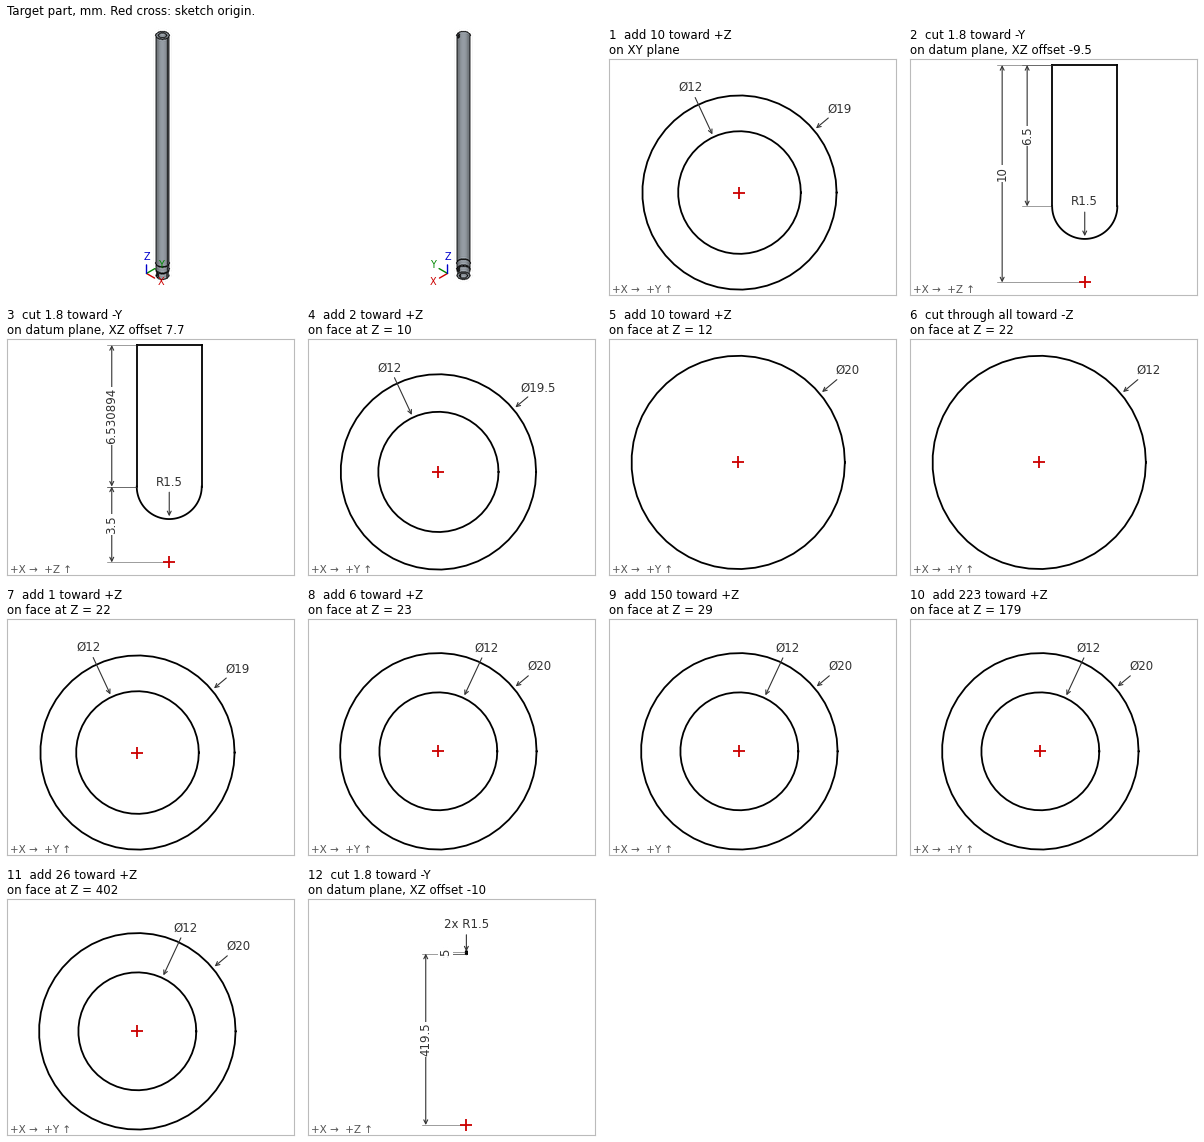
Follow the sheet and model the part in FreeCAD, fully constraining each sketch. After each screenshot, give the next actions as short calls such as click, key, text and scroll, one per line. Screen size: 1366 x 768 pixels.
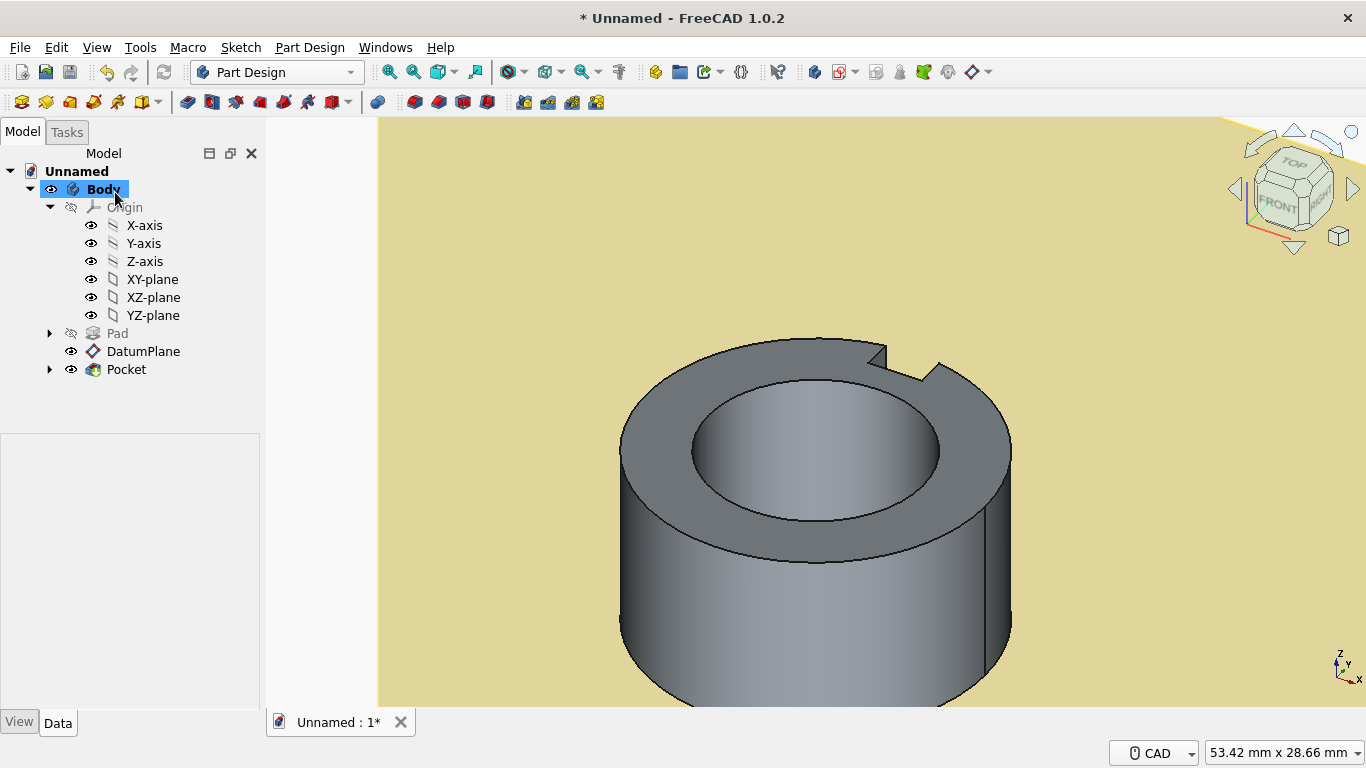
click(116, 351)
key(space)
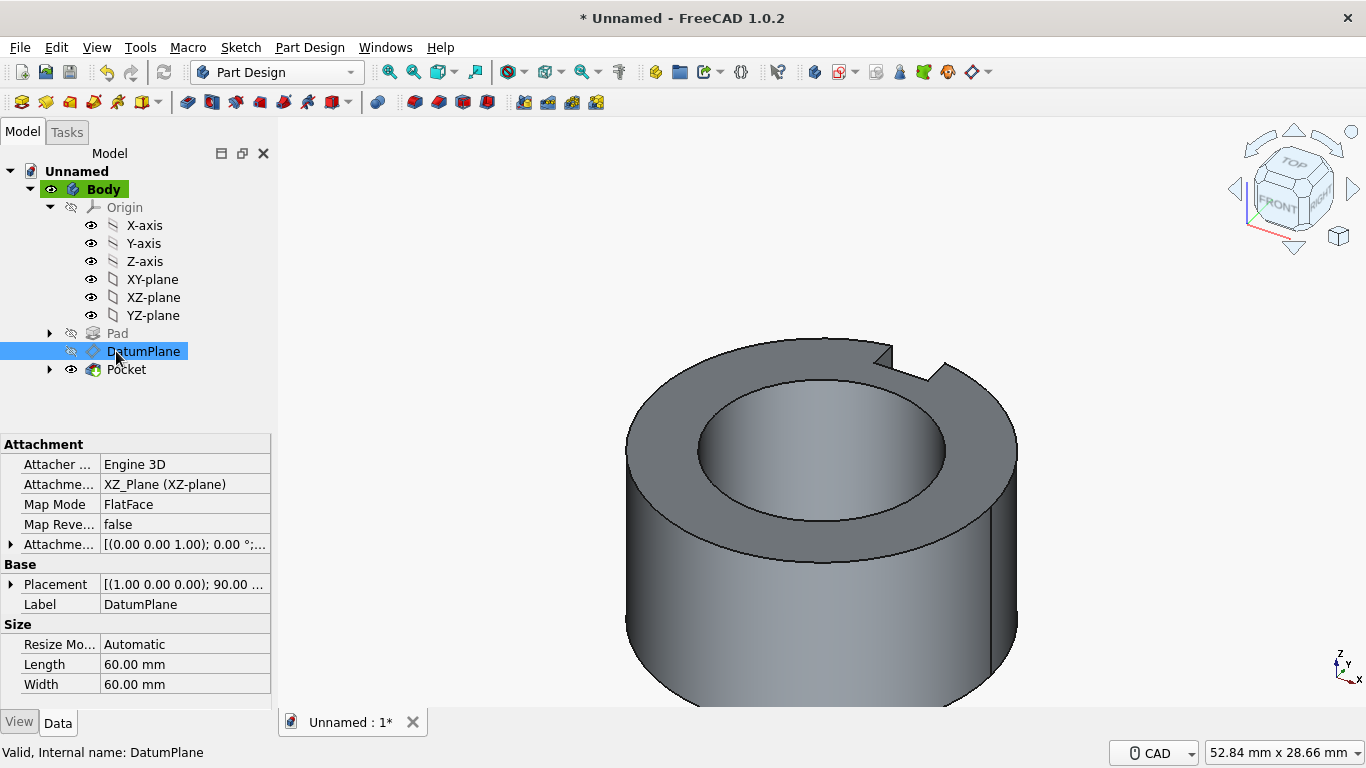
click(390, 72)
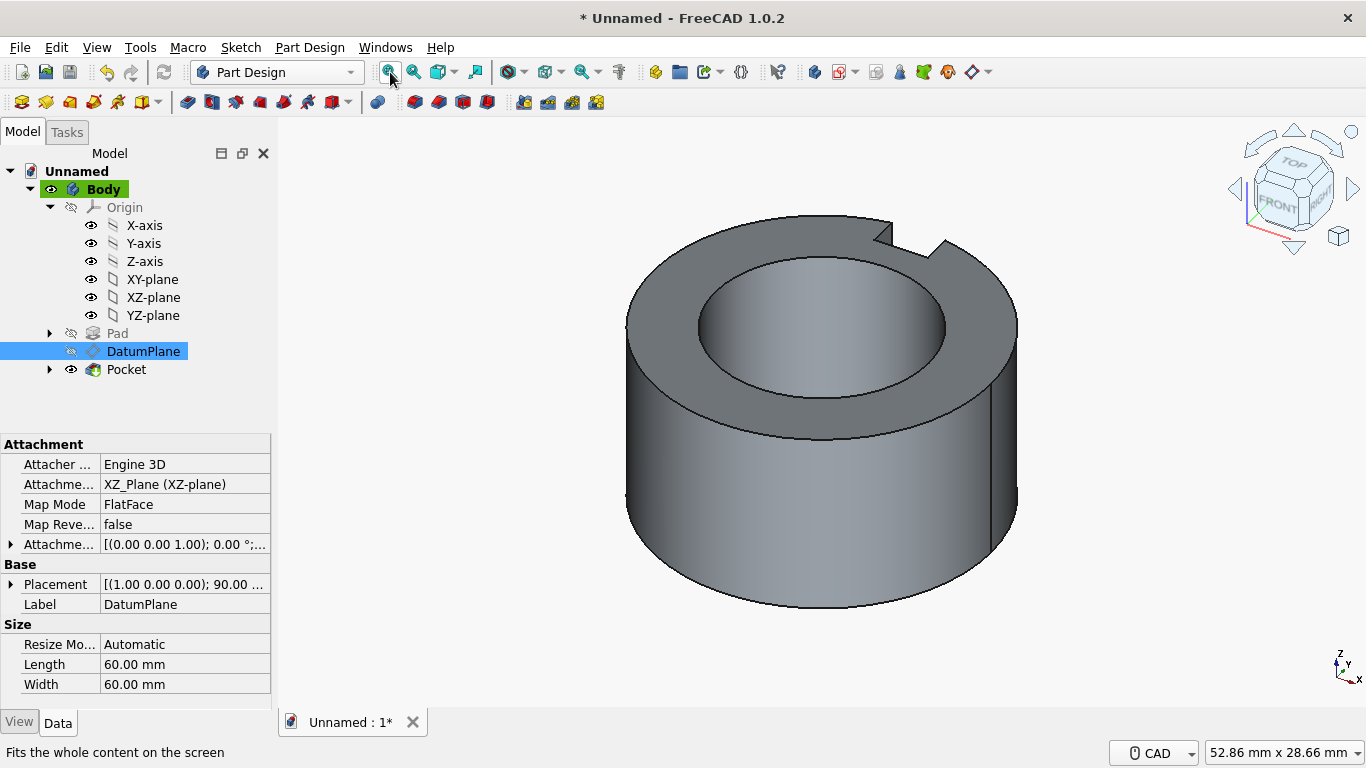
click(136, 297)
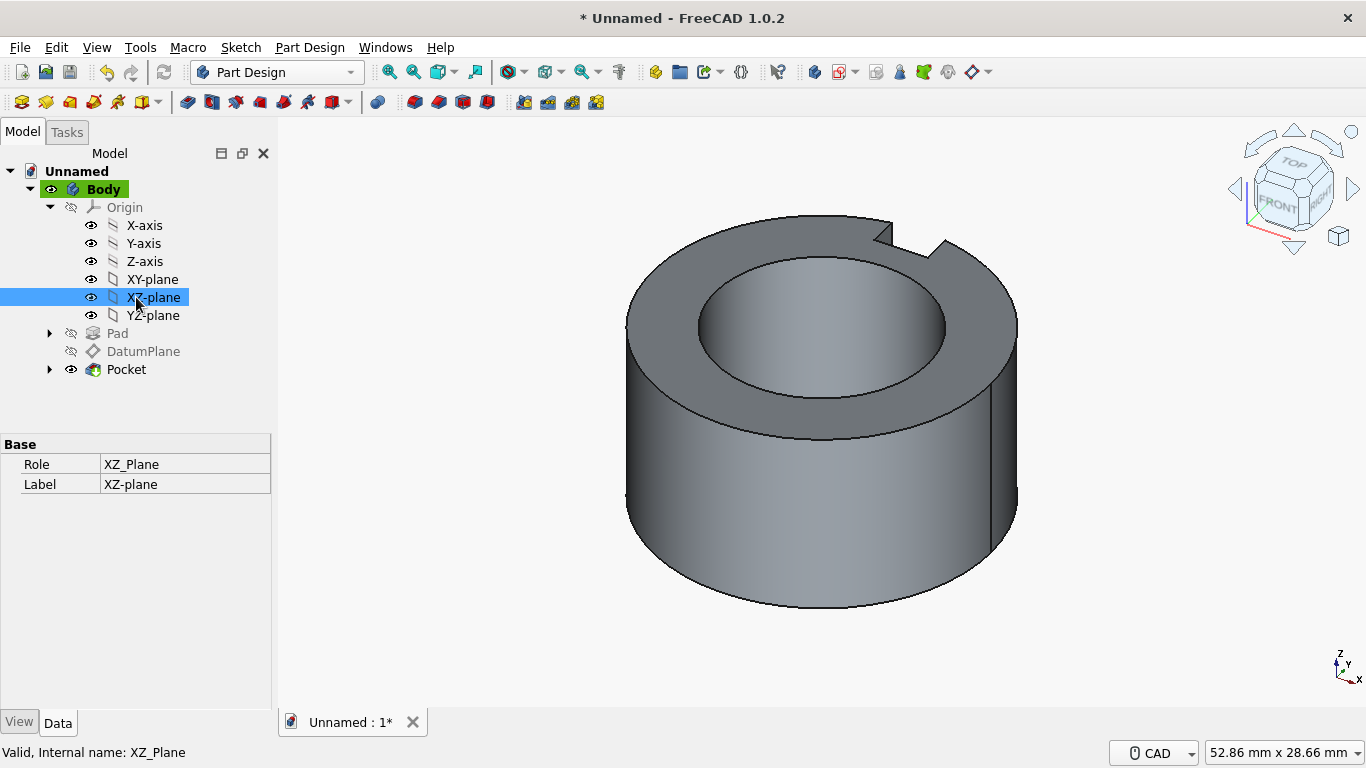
click(972, 72)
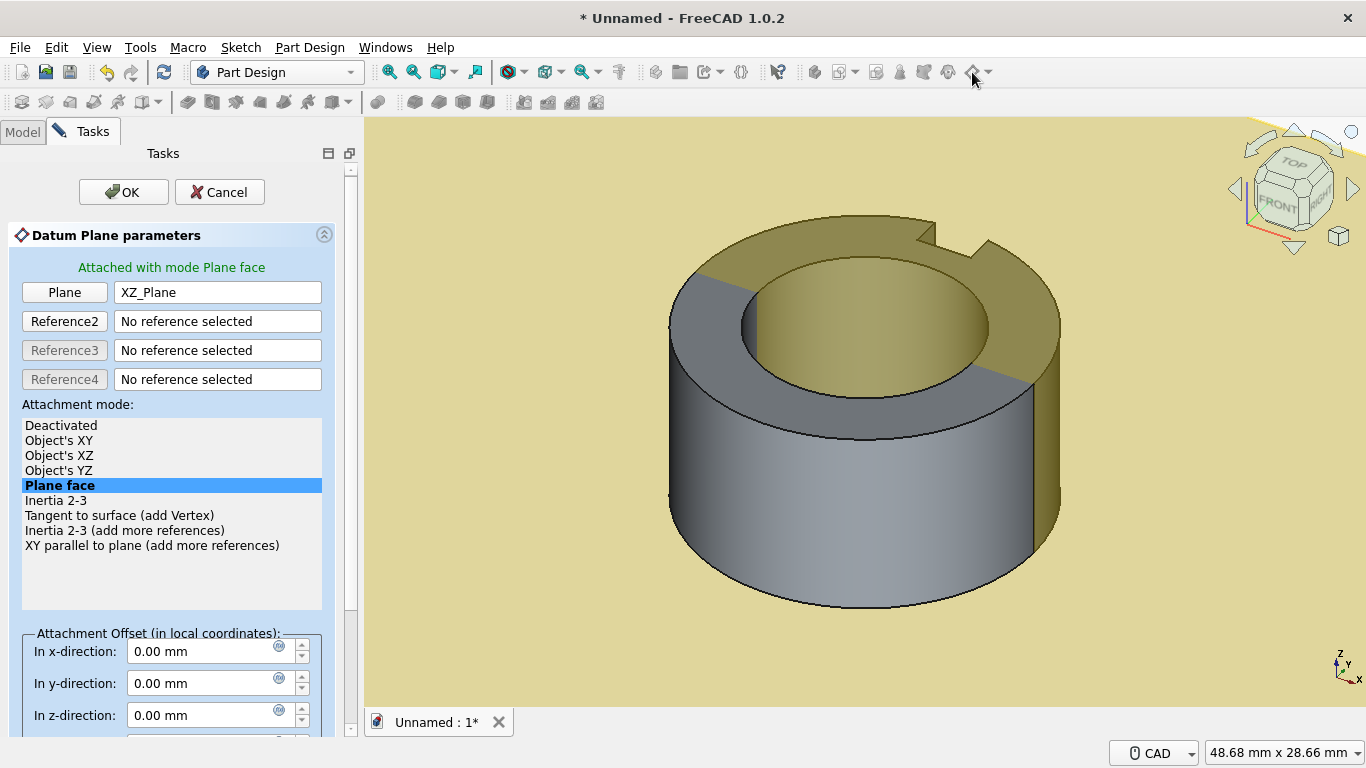
triple_click(210, 715)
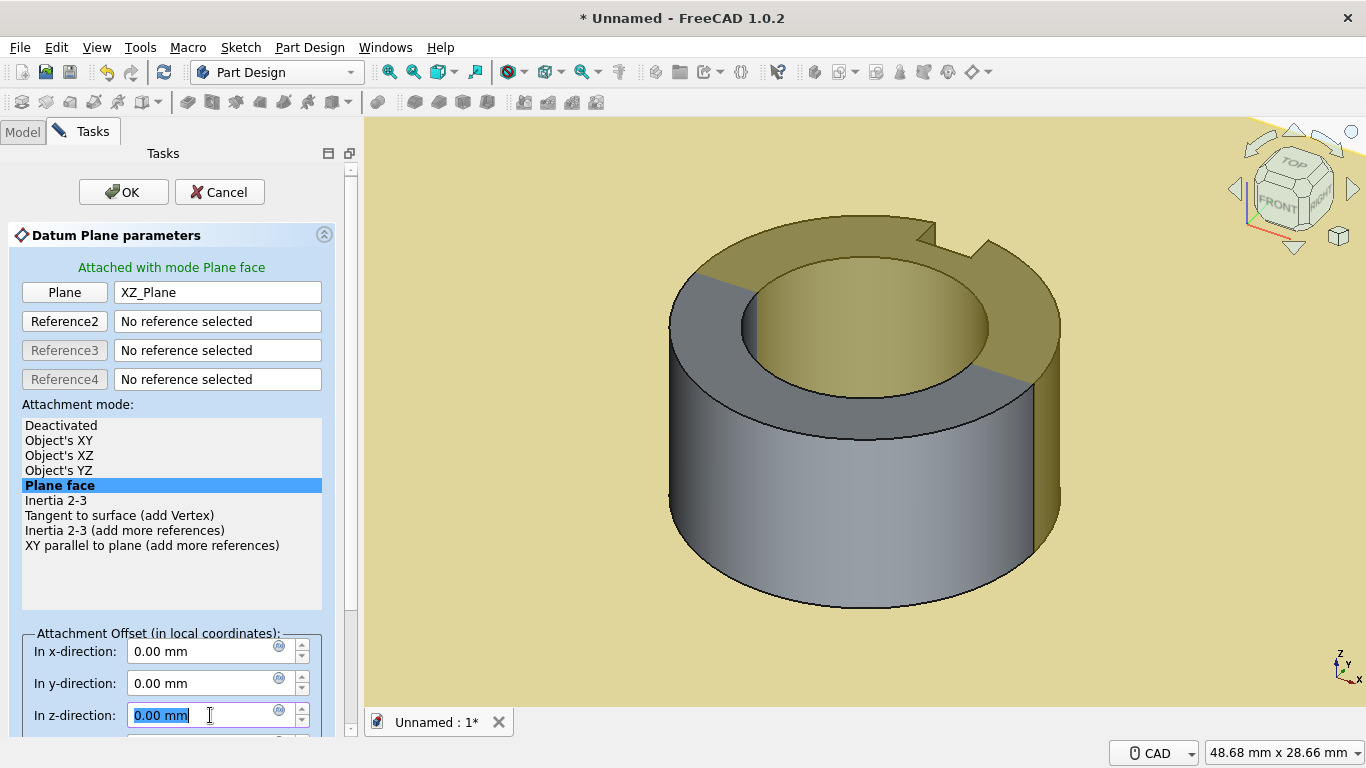
text(7.7)
key(Tab)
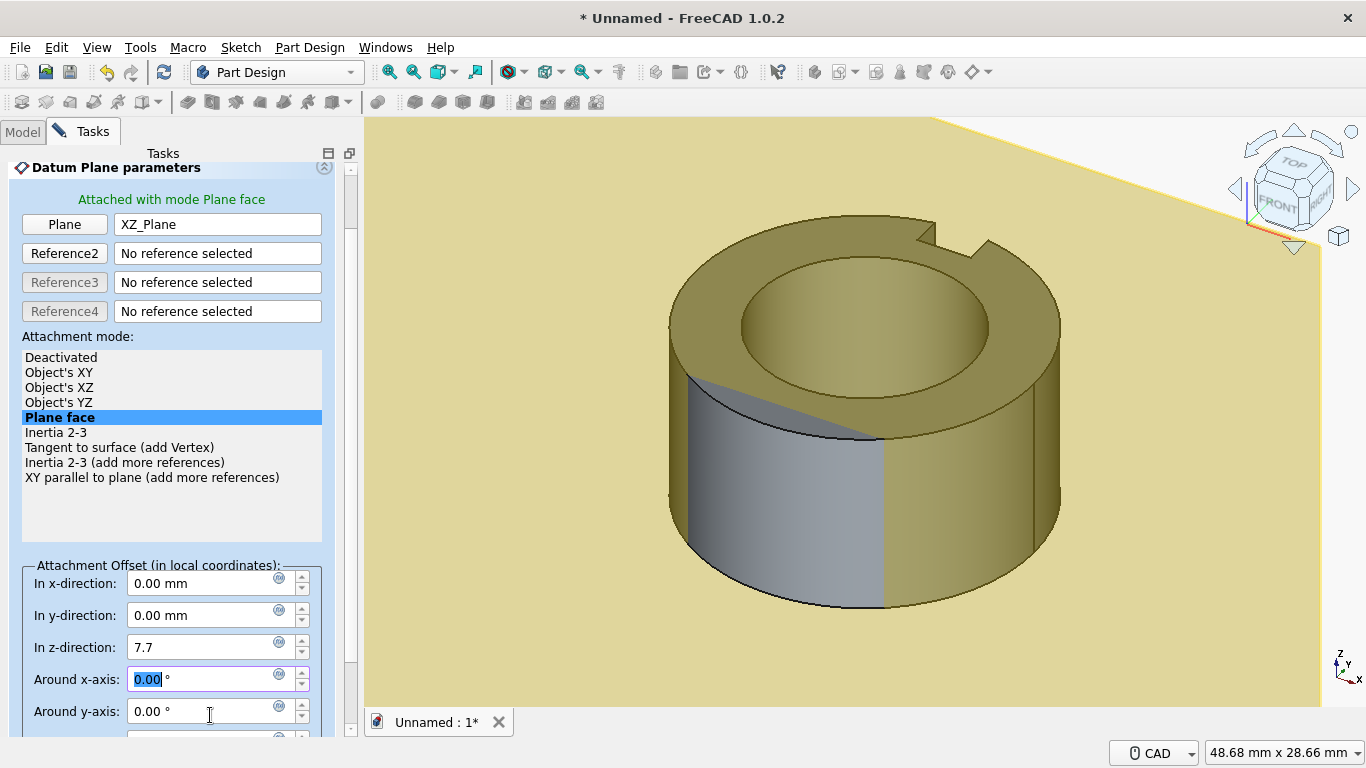
scroll(351, 450, up, 2)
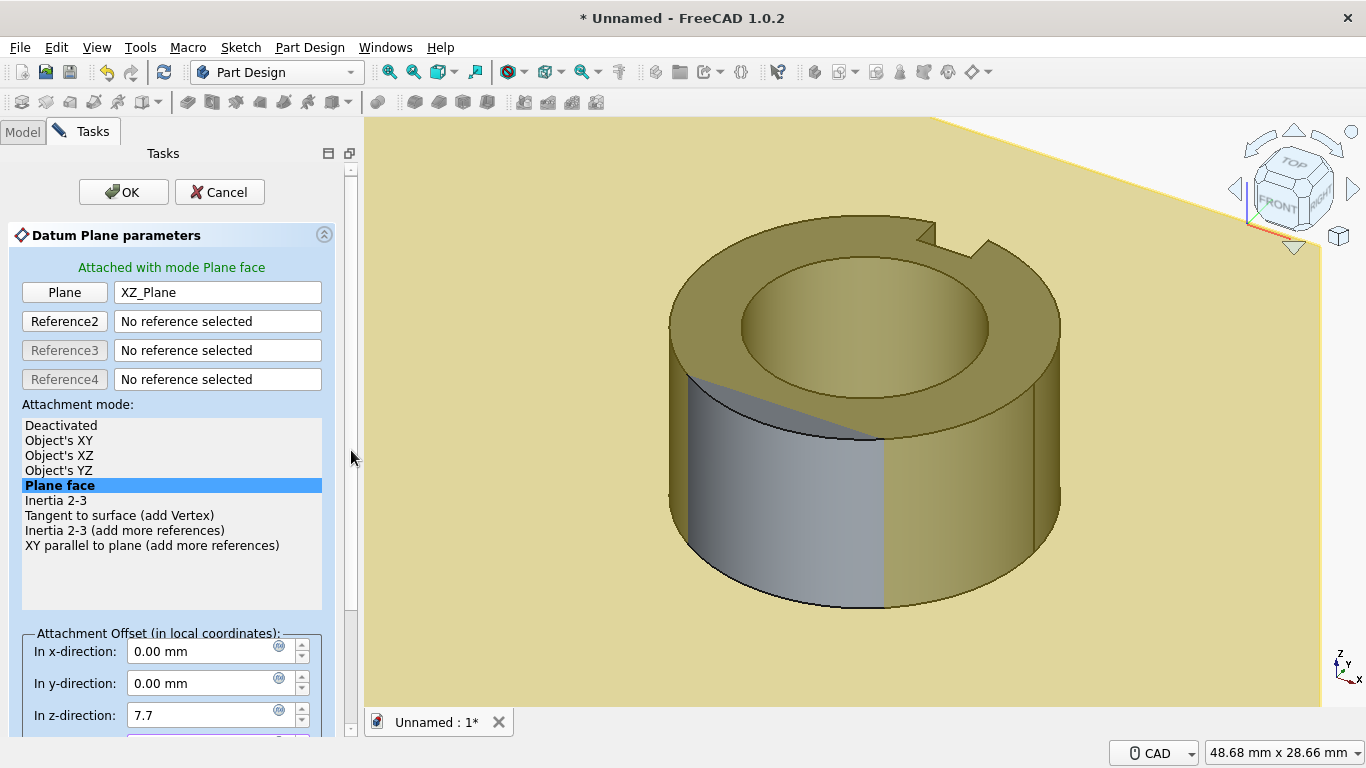
click(124, 192)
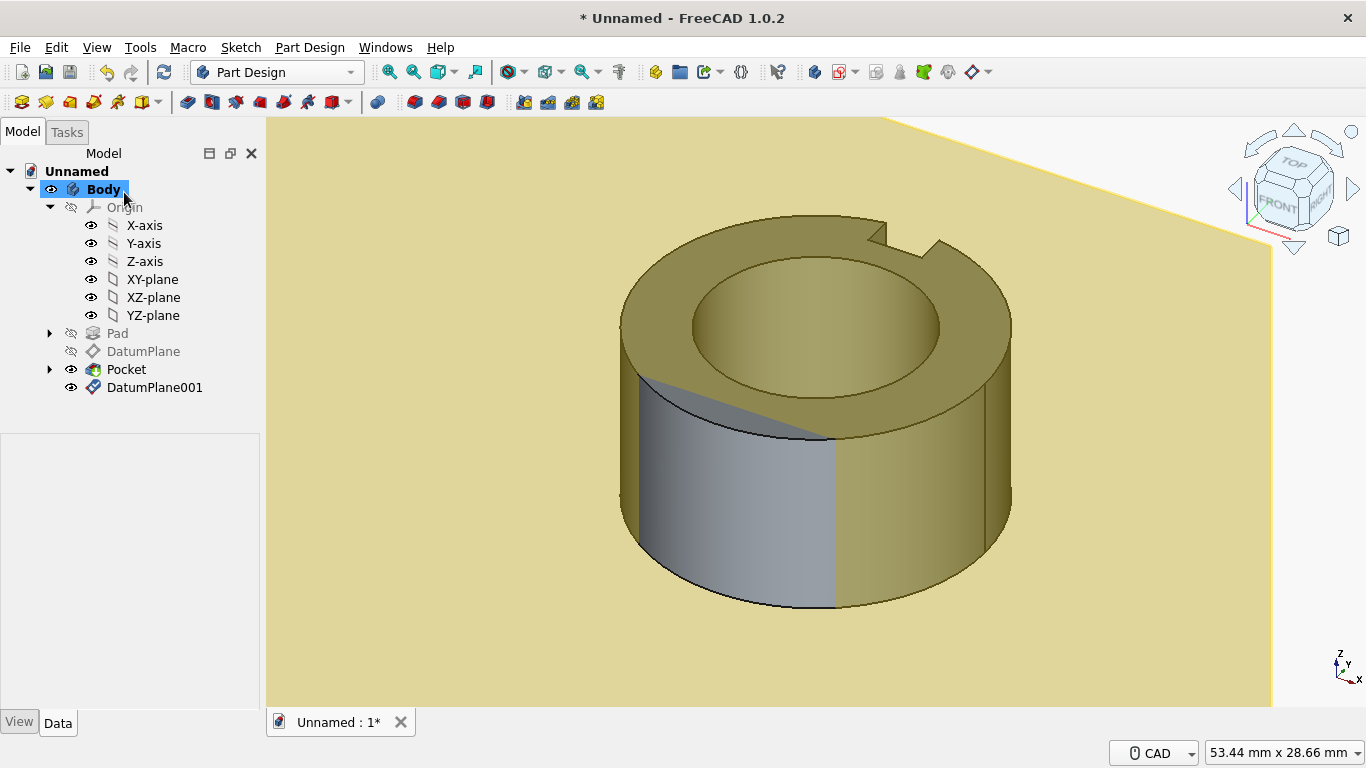
click(116, 387)